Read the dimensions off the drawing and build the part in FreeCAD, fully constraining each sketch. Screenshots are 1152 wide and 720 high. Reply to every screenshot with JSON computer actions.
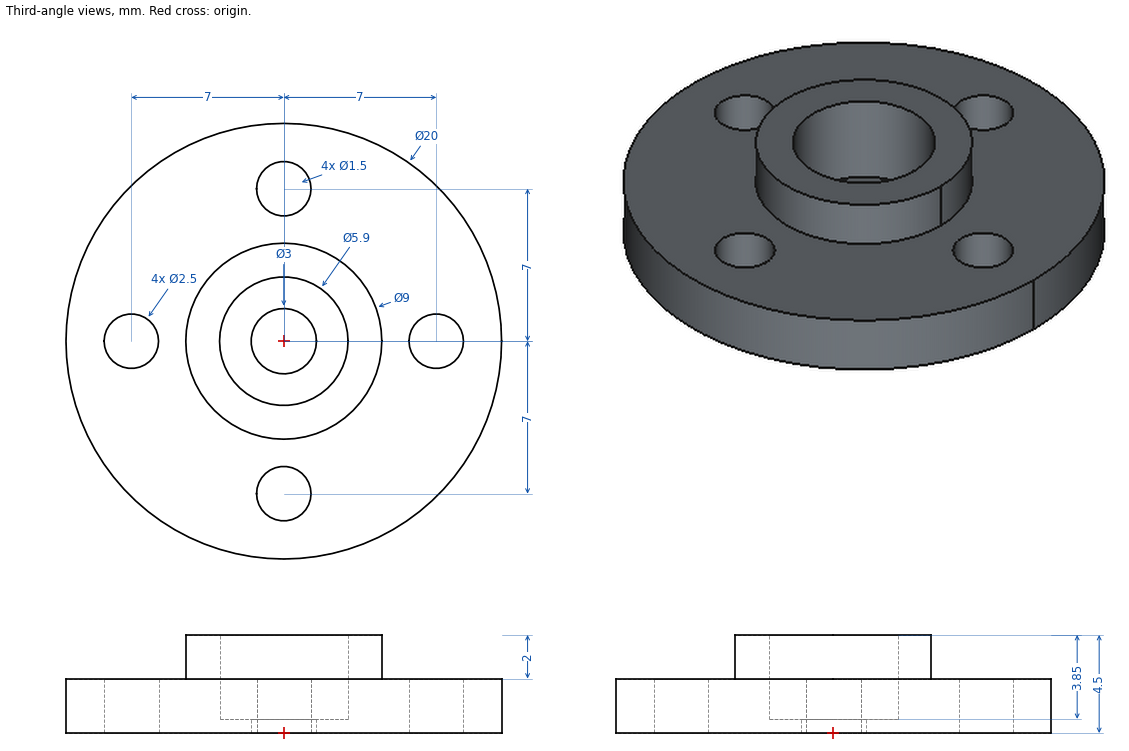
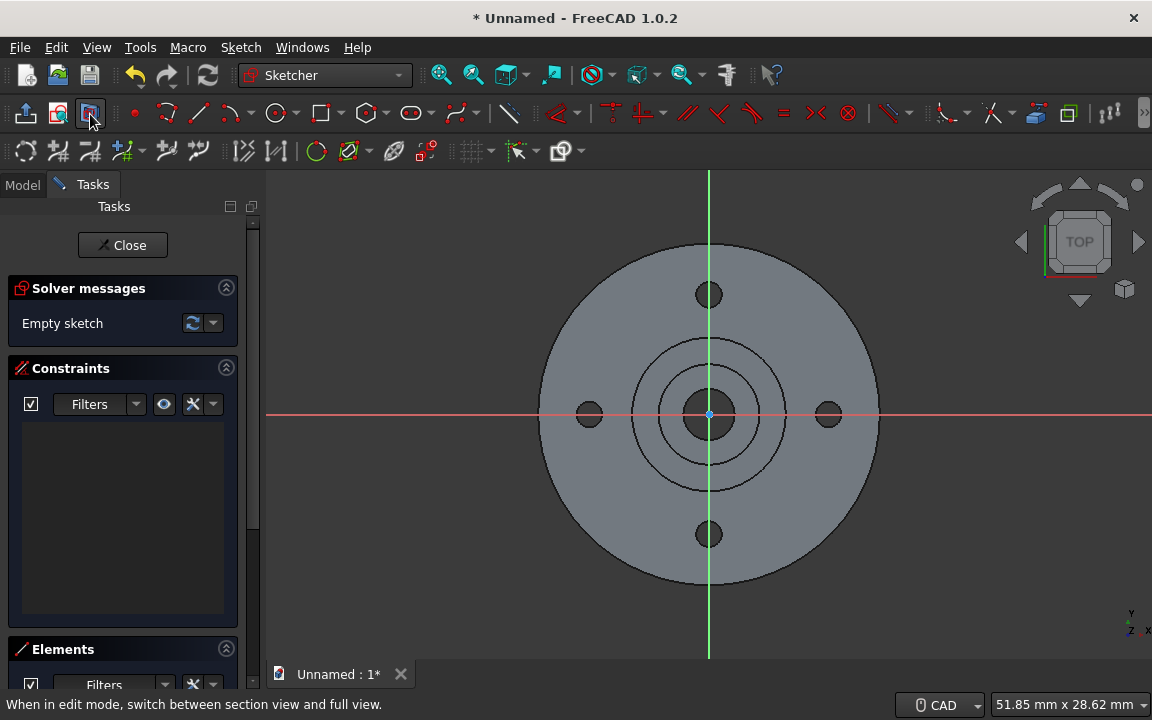
{"action": "key", "text": "g c"}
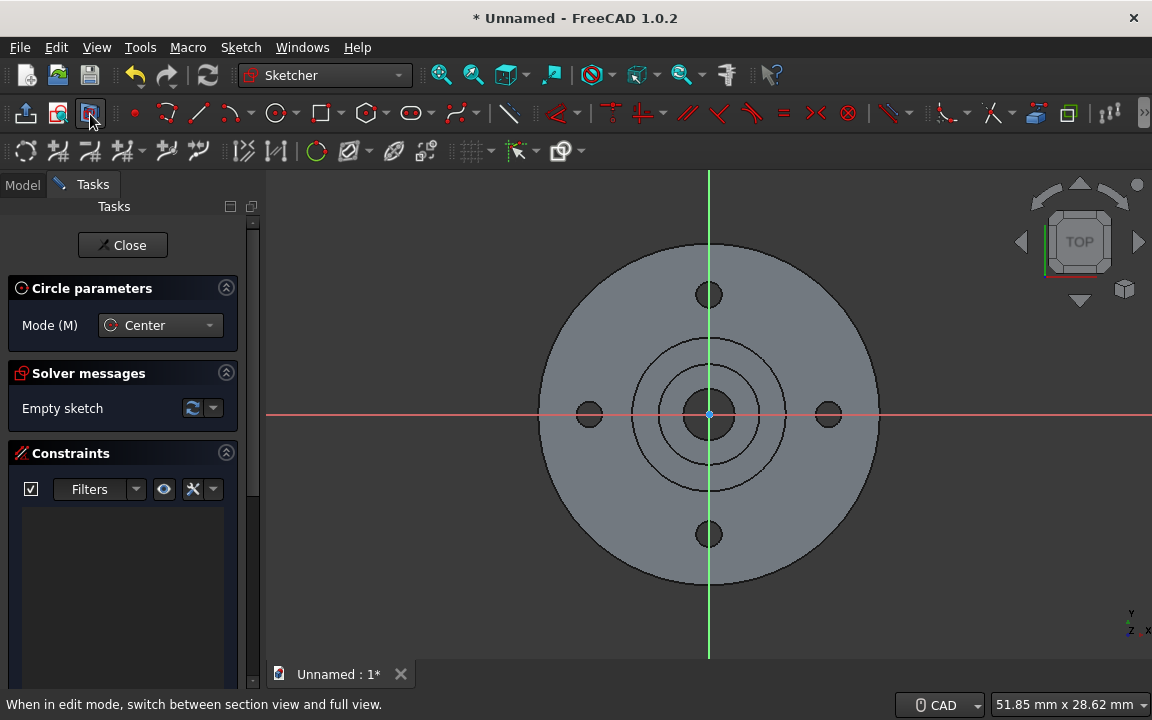
{"action": "left_click", "coordinate": [589, 414]}
{"action": "left_click", "coordinate": [604, 399]}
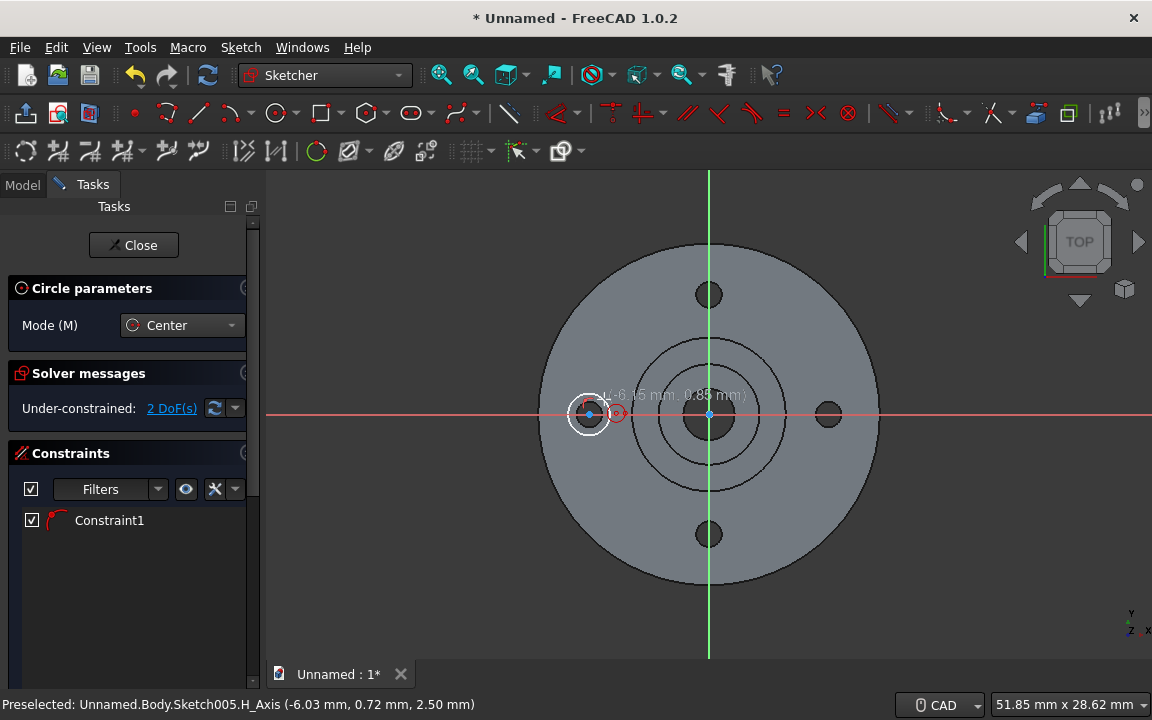
{"action": "left_click", "coordinate": [709, 295]}
{"action": "left_click", "coordinate": [724, 280]}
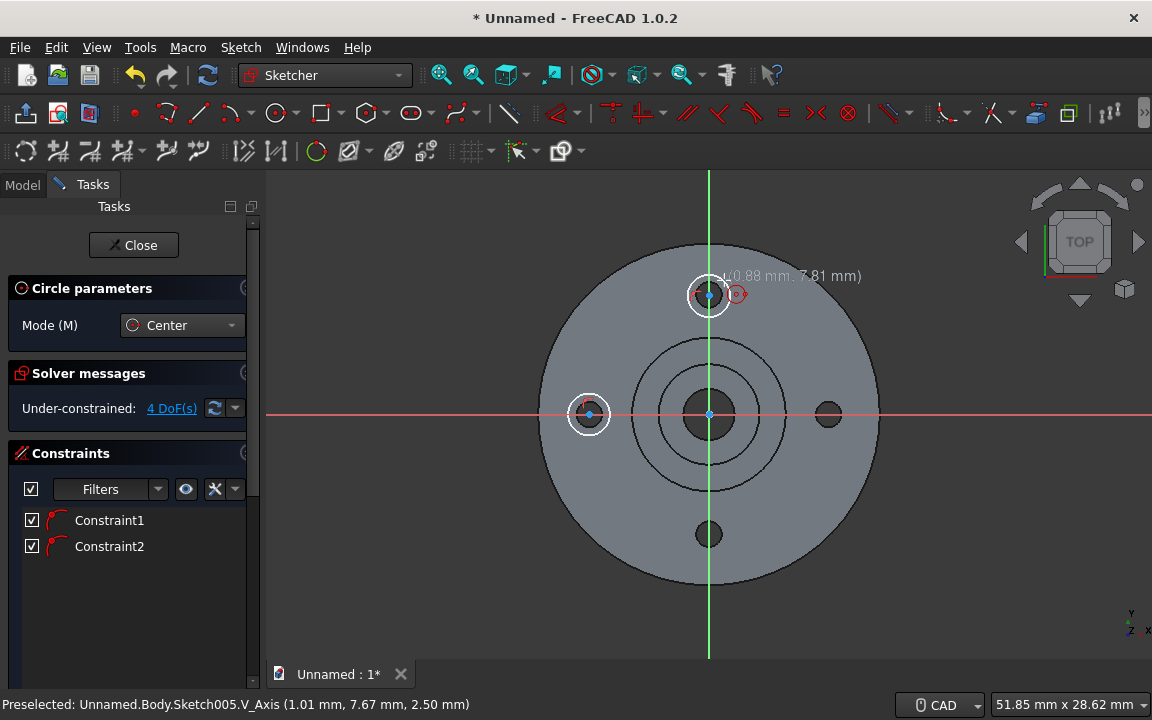
{"action": "left_click", "coordinate": [829, 414]}
{"action": "left_click", "coordinate": [844, 399]}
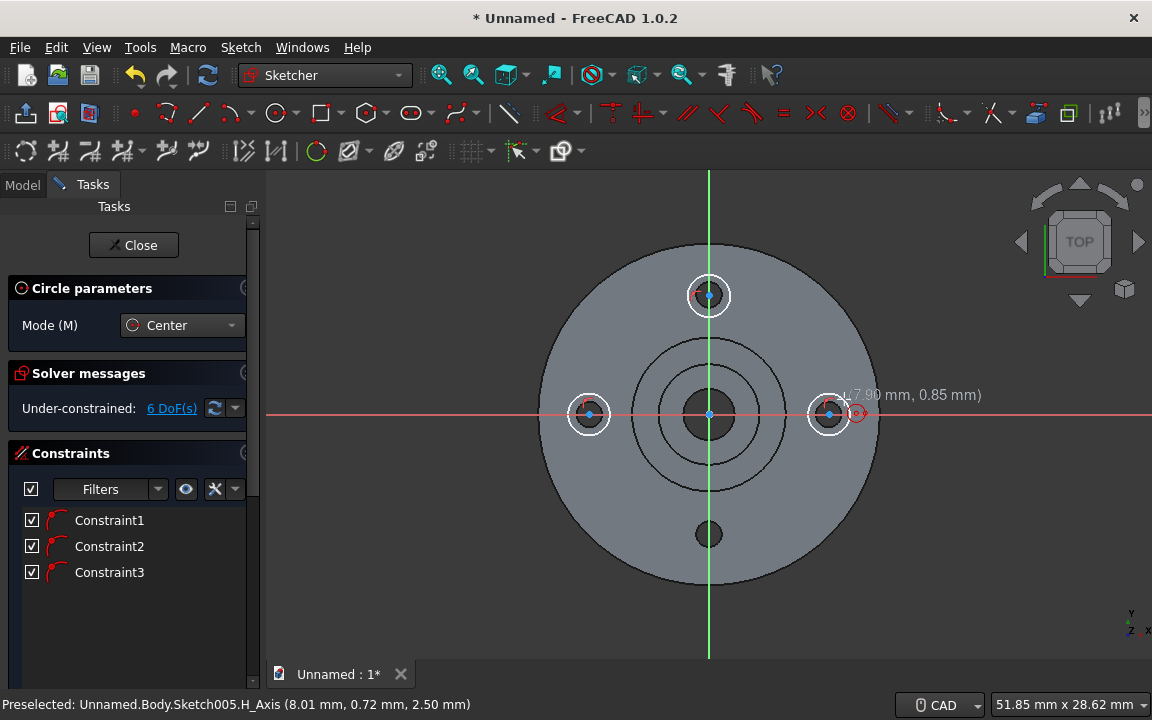
{"action": "left_click", "coordinate": [709, 534]}
{"action": "left_click", "coordinate": [724, 519]}
{"action": "key", "text": "Escape"}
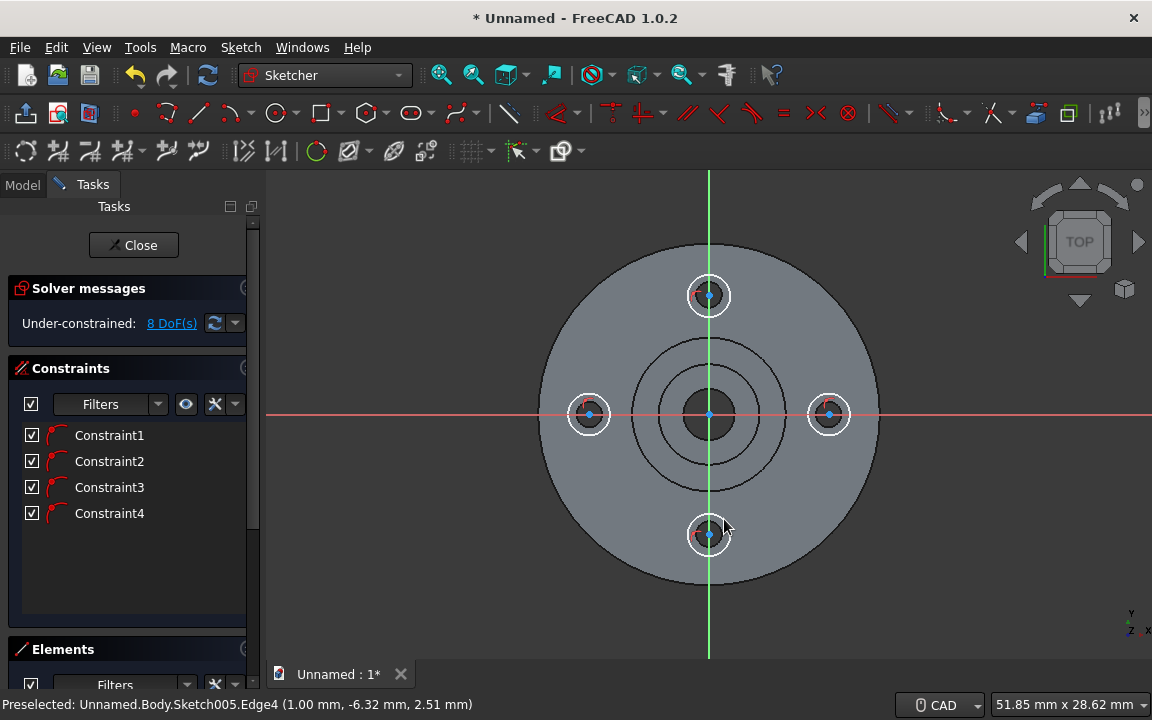
{"action": "left_click", "coordinate": [604, 400]}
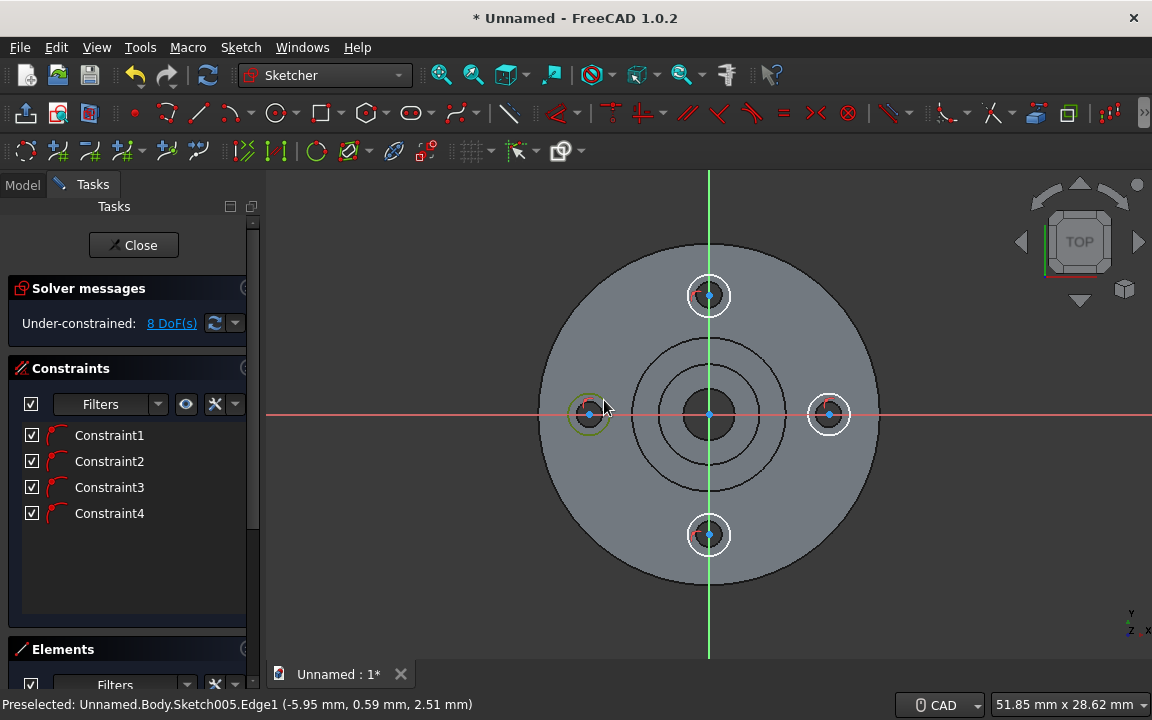
{"action": "left_click", "coordinate": [724, 281]}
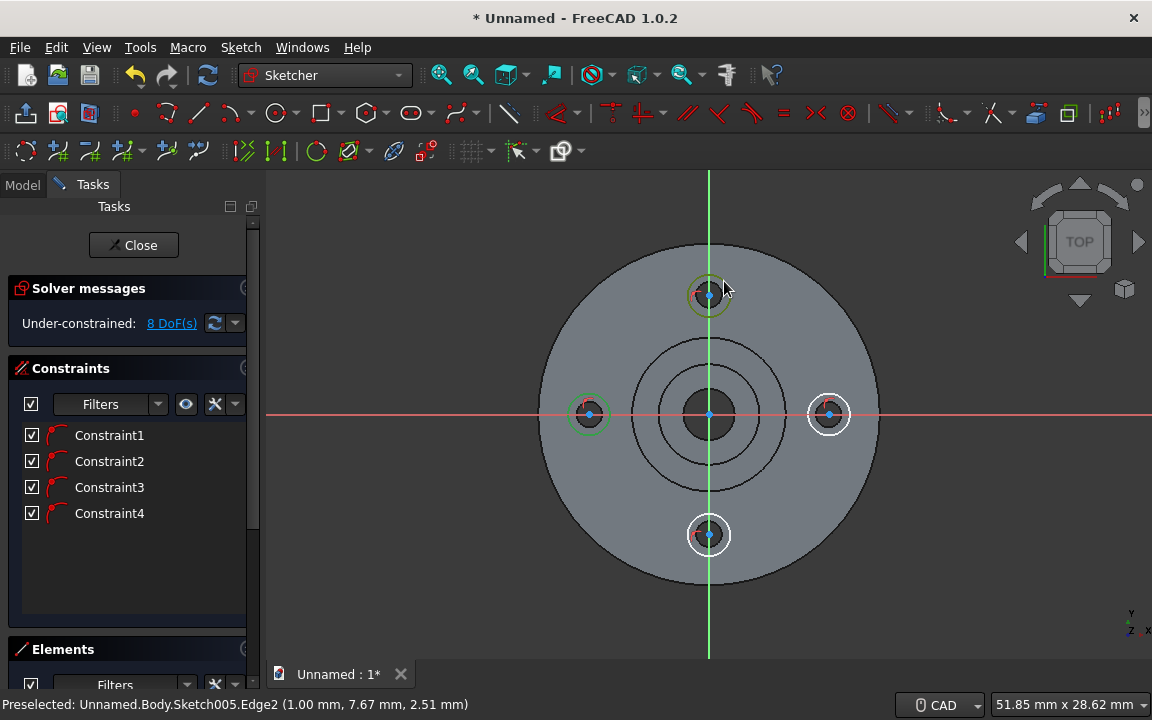
{"action": "left_click", "coordinate": [844, 400]}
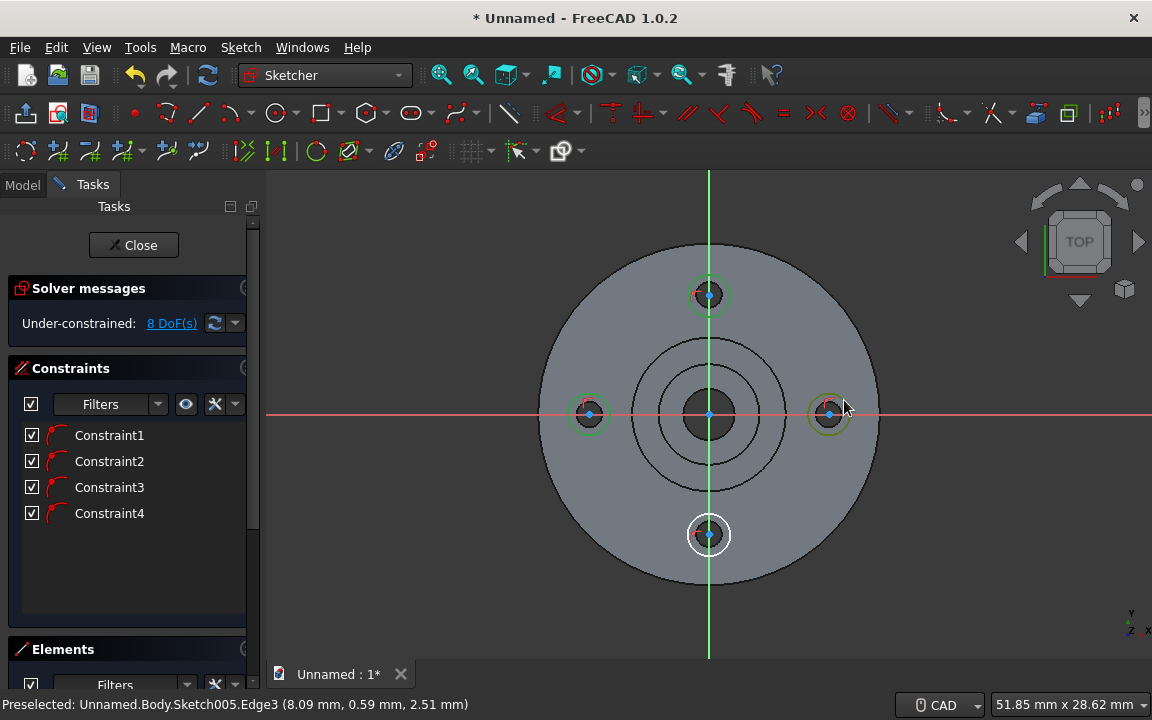
{"action": "left_click", "coordinate": [724, 520]}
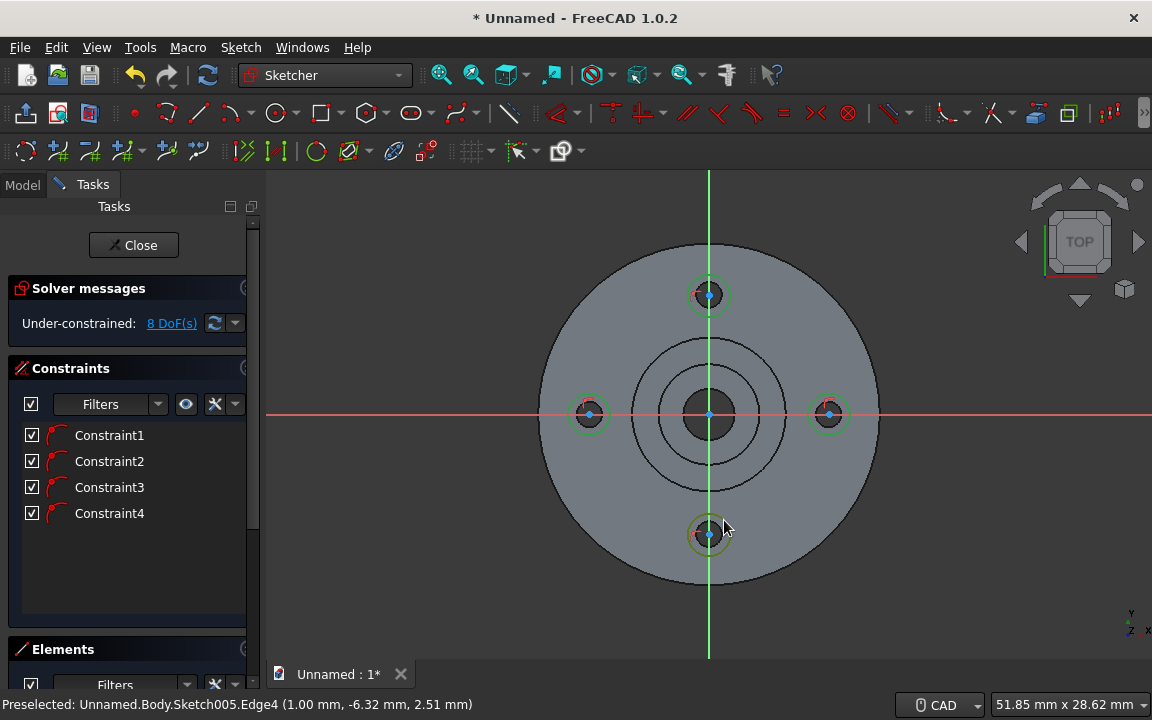
{"action": "left_click", "coordinate": [784, 114]}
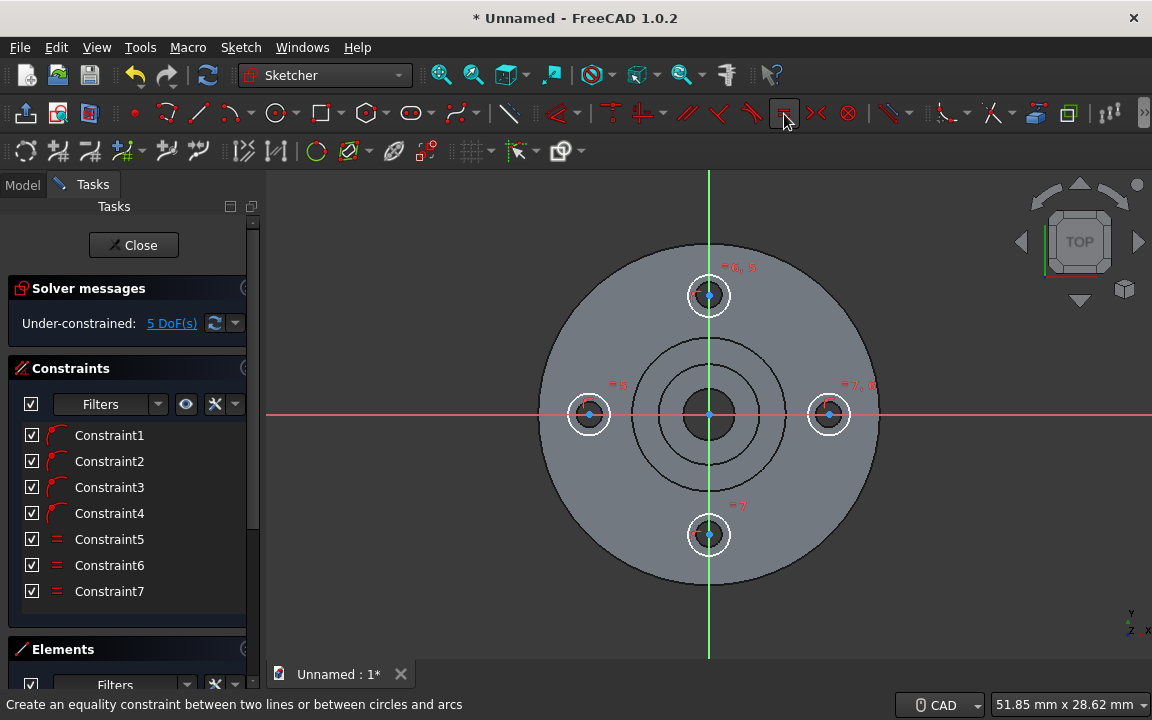
{"action": "key", "text": "d"}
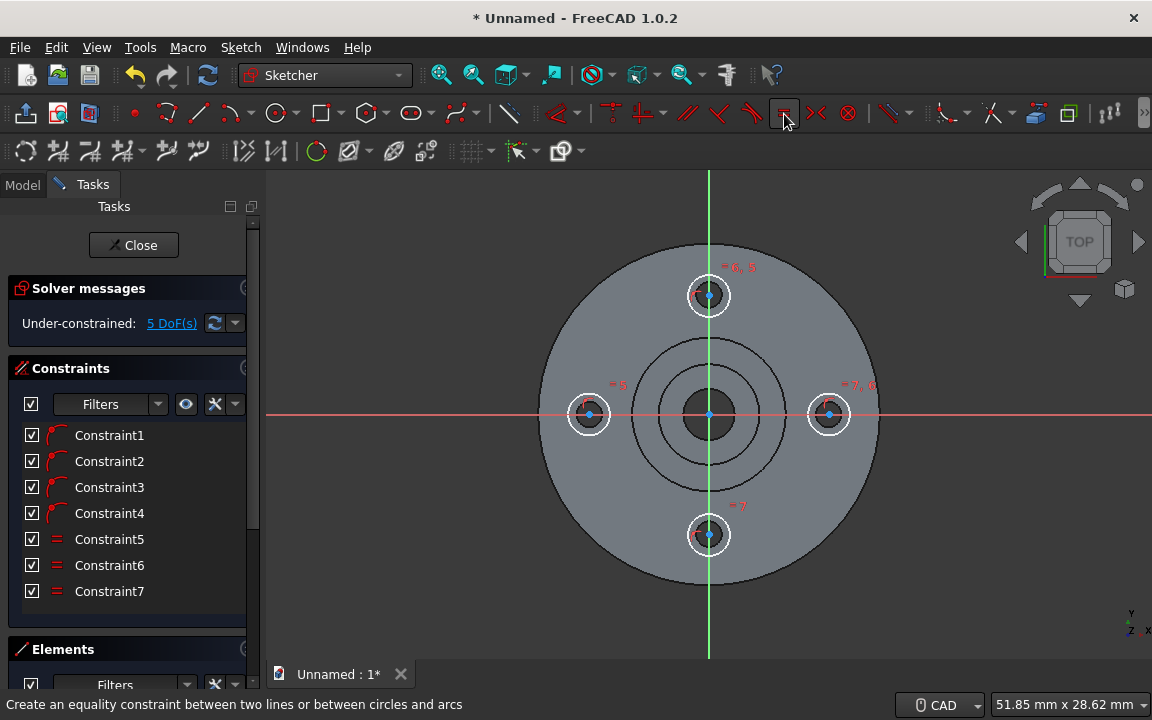
{"action": "left_click", "coordinate": [604, 400]}
{"action": "left_click", "coordinate": [627, 378]}